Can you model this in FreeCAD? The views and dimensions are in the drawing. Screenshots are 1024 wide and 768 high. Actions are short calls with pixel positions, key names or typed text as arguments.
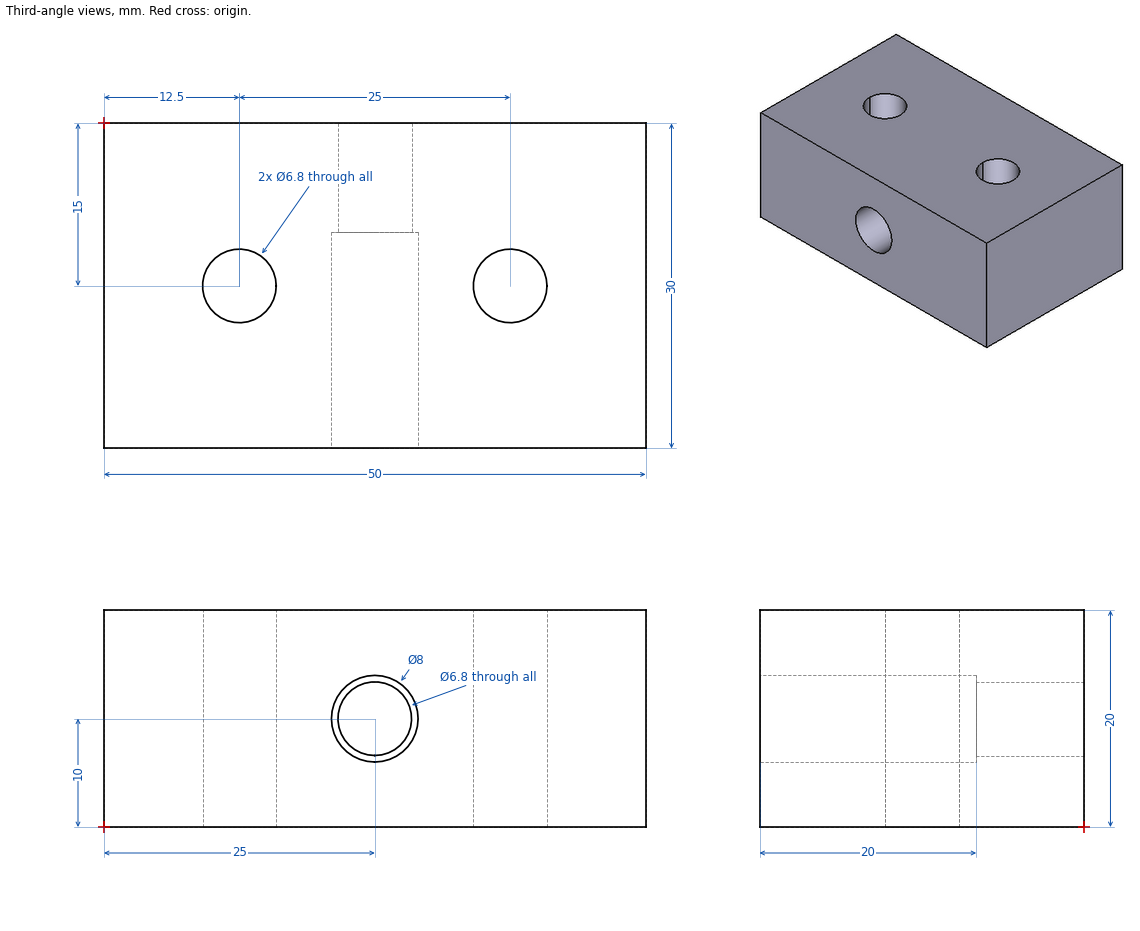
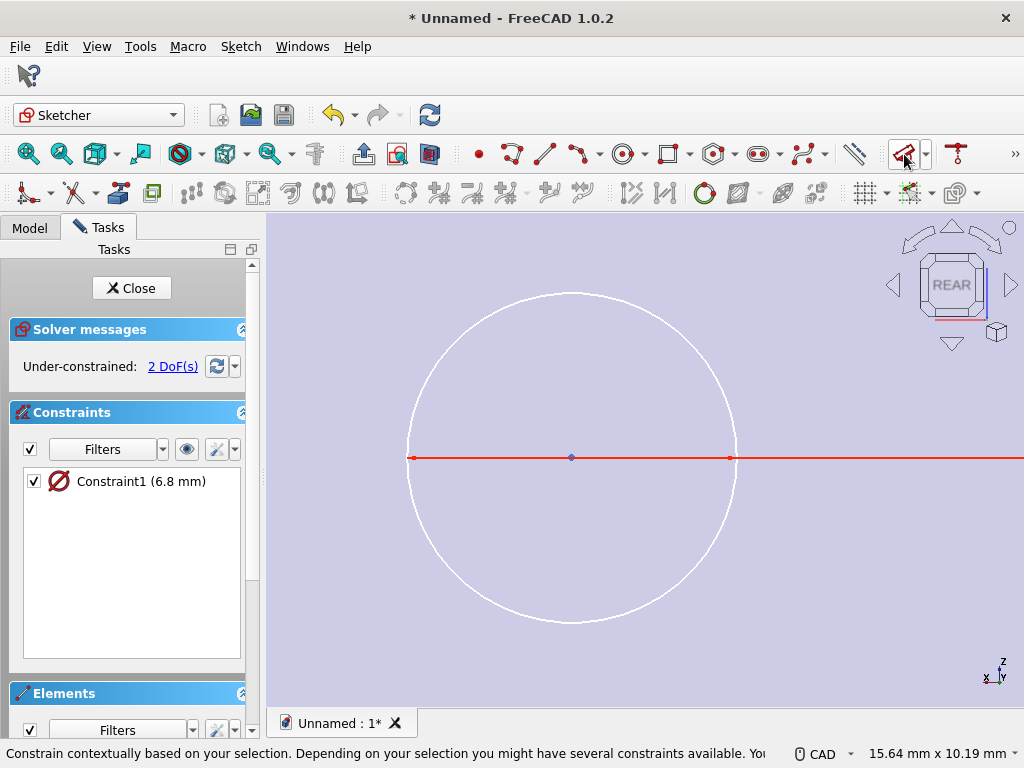
click(572, 458)
click(716, 424)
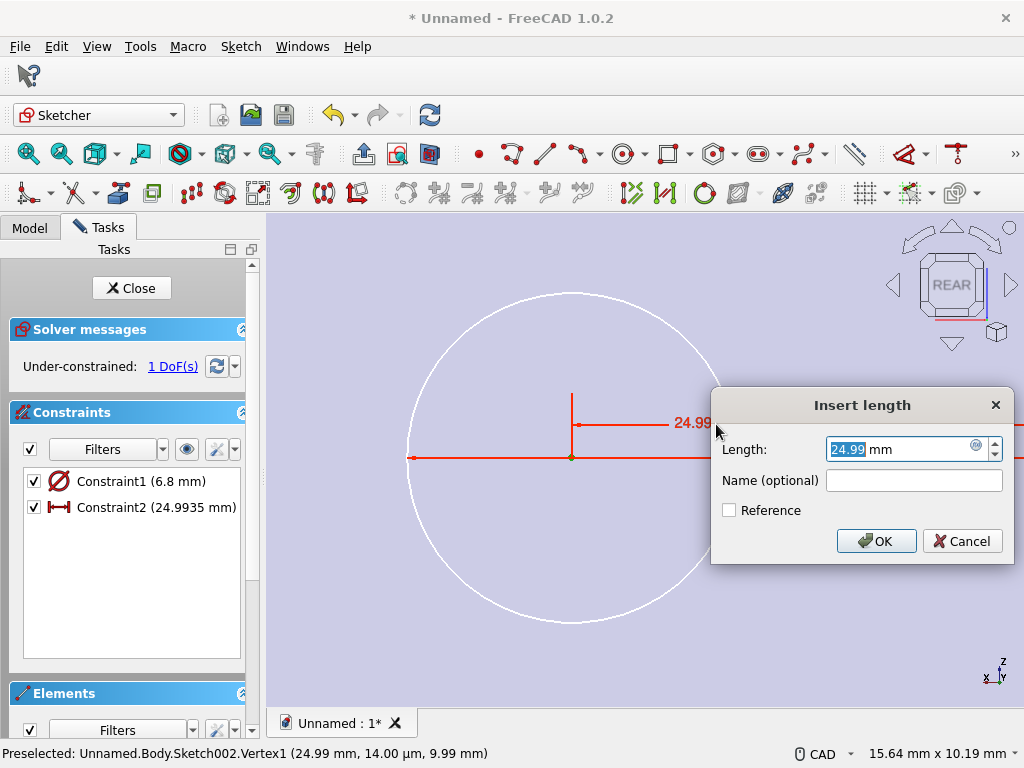
text(25)
key(Return)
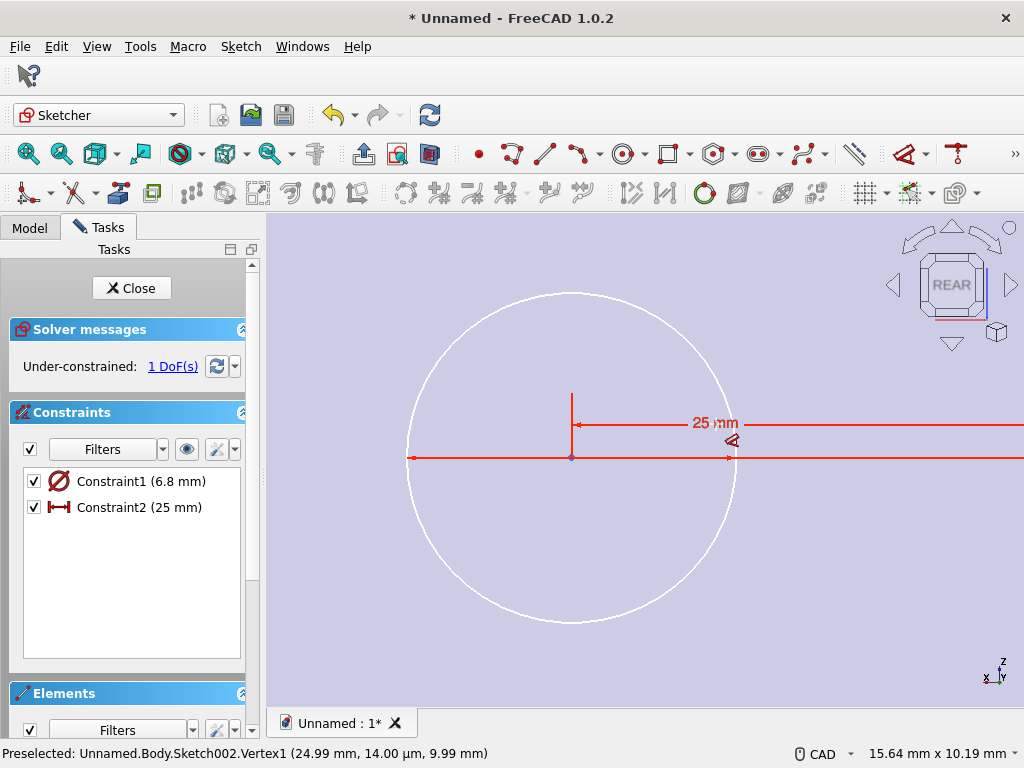
click(572, 458)
click(538, 568)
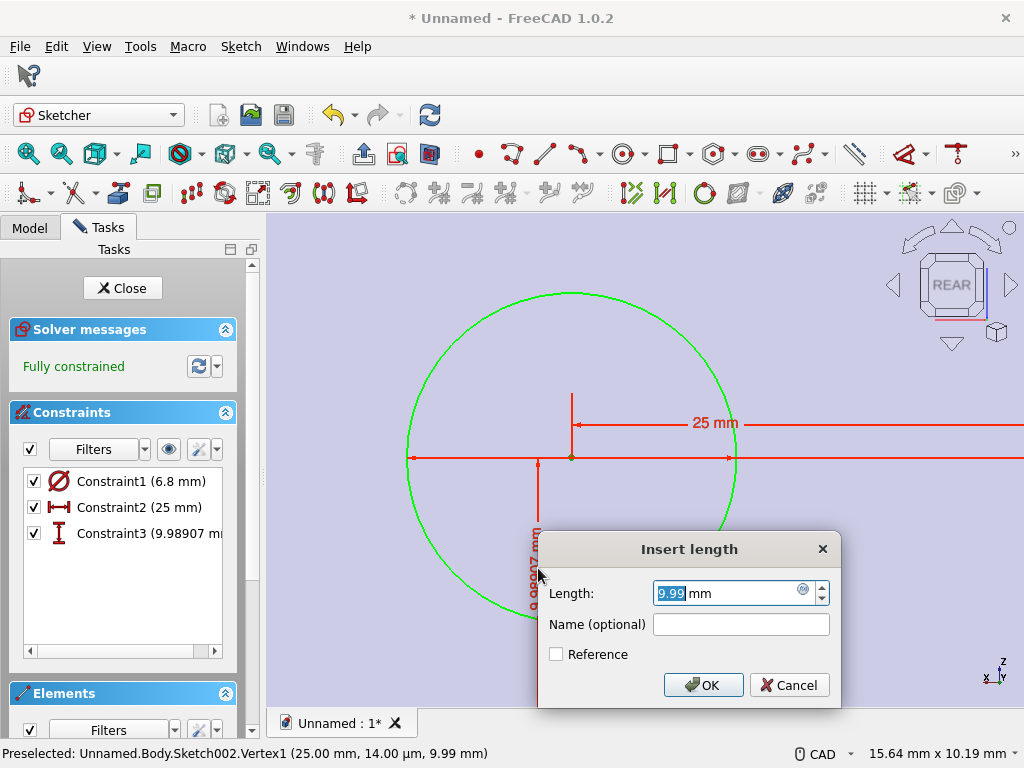
text(10)
key(Return)
key(Escape)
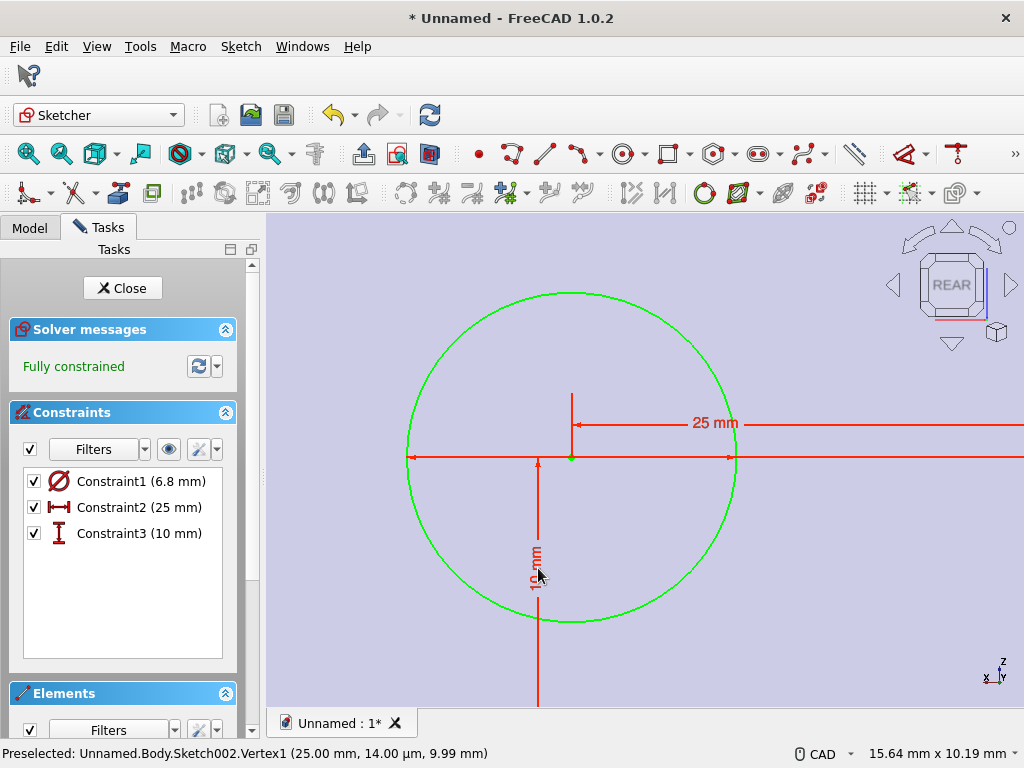
click(123, 288)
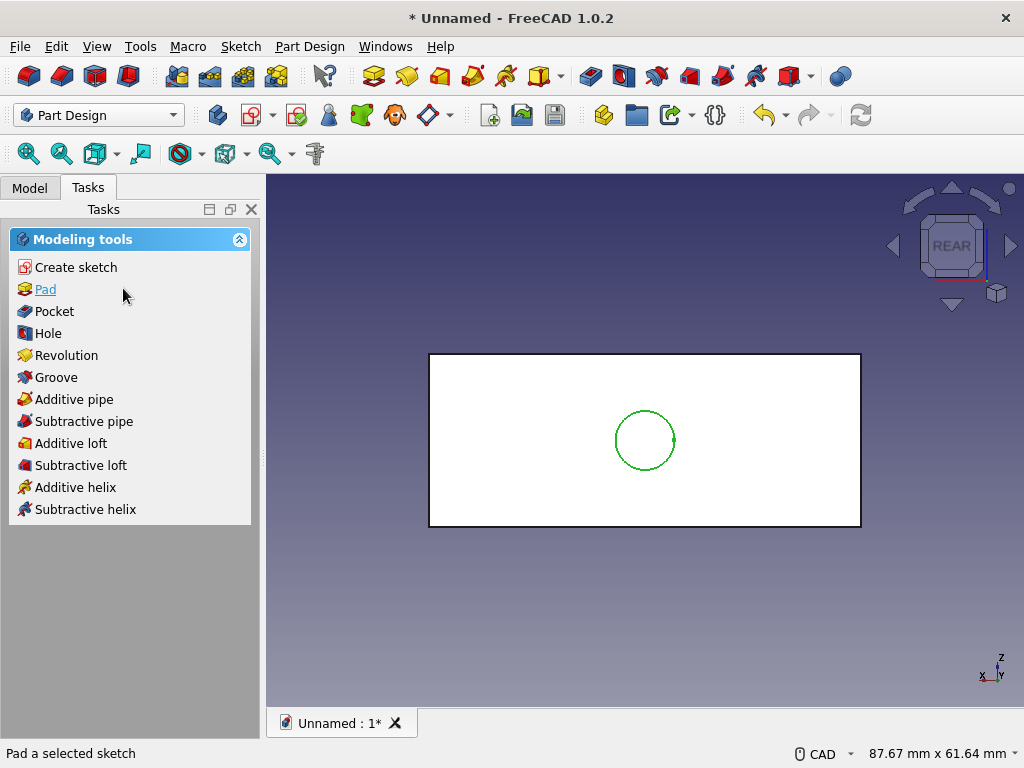
click(624, 76)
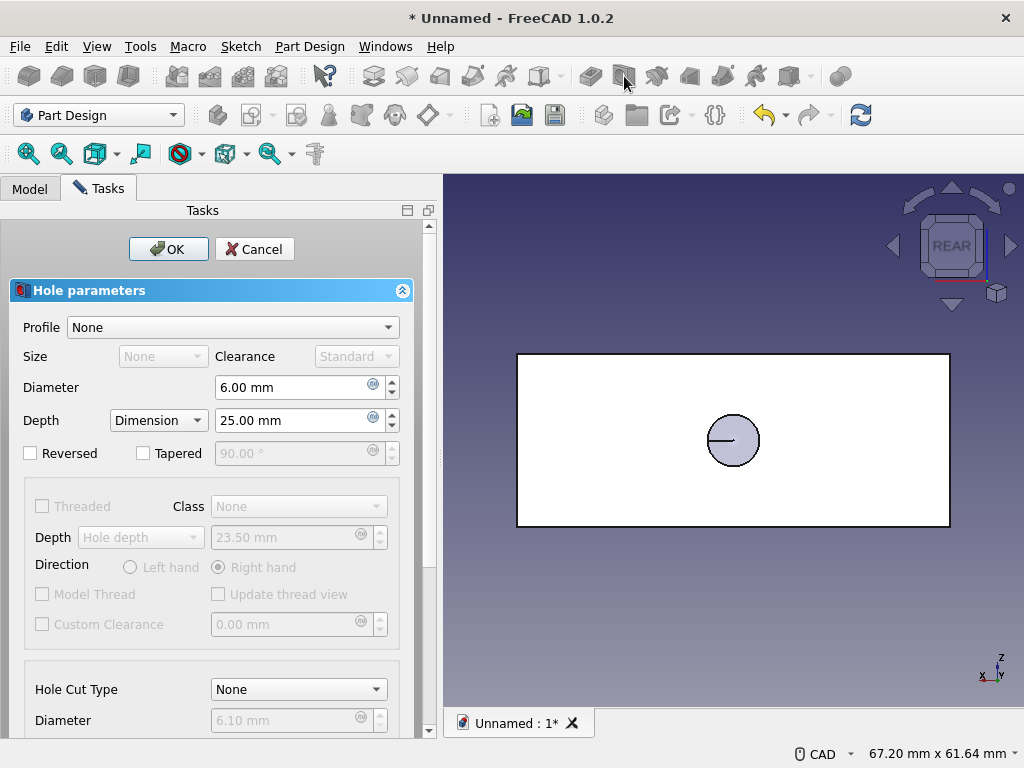
triple_click(300, 388)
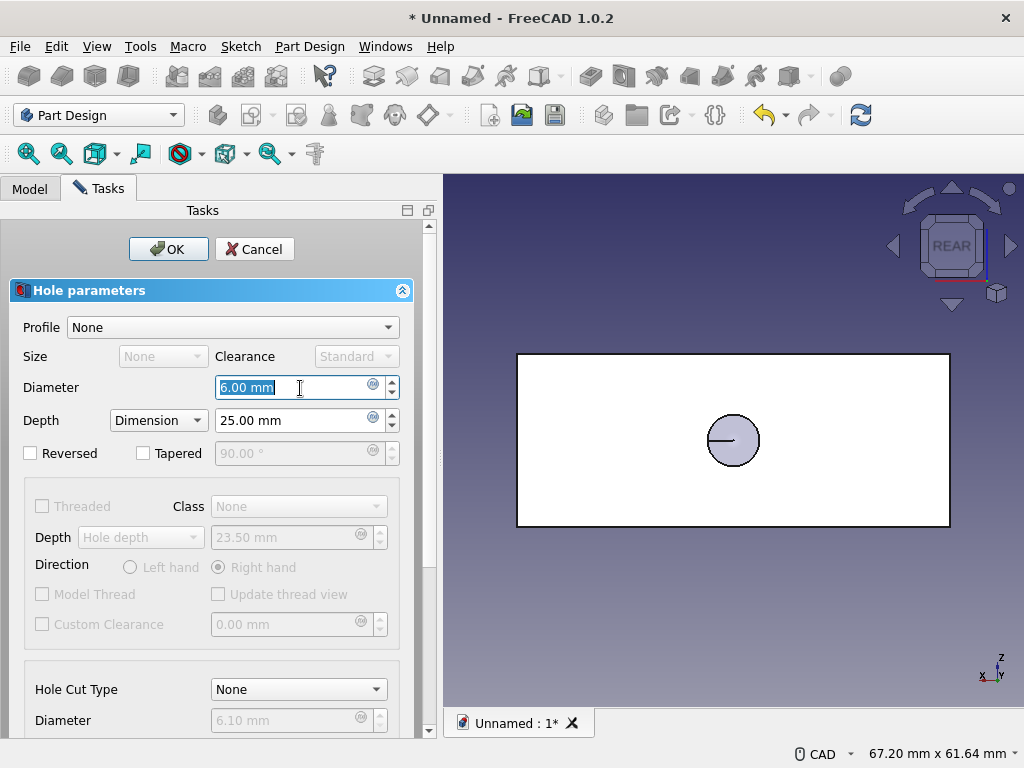
text(6.8)
key(Tab)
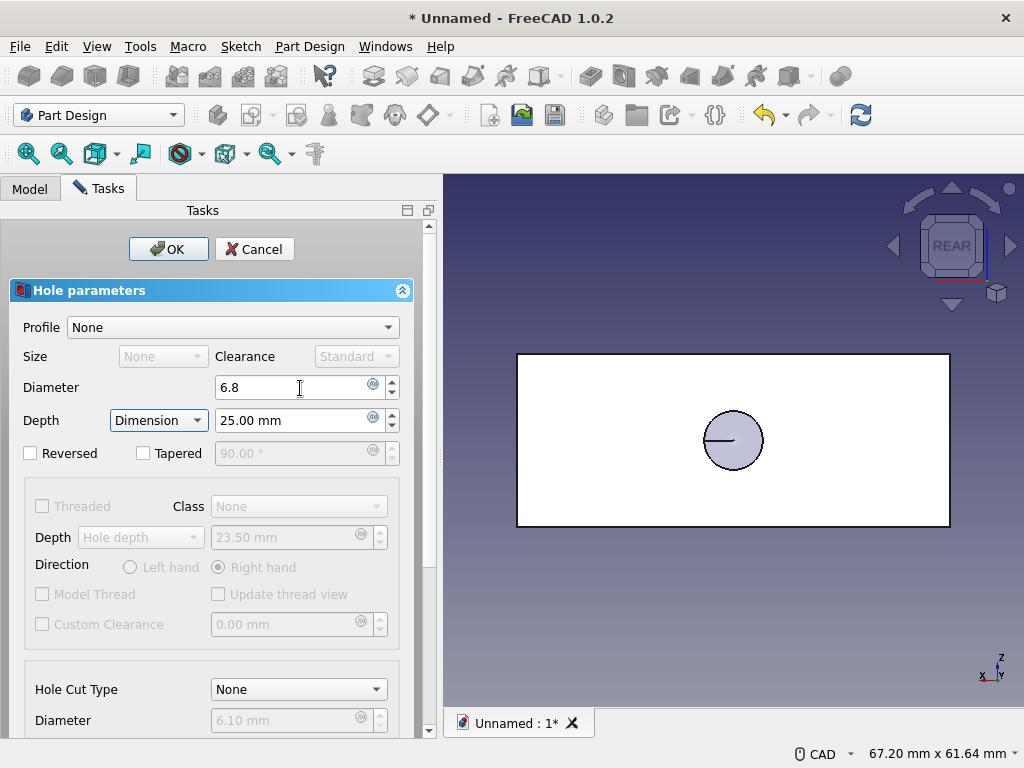
click(160, 420)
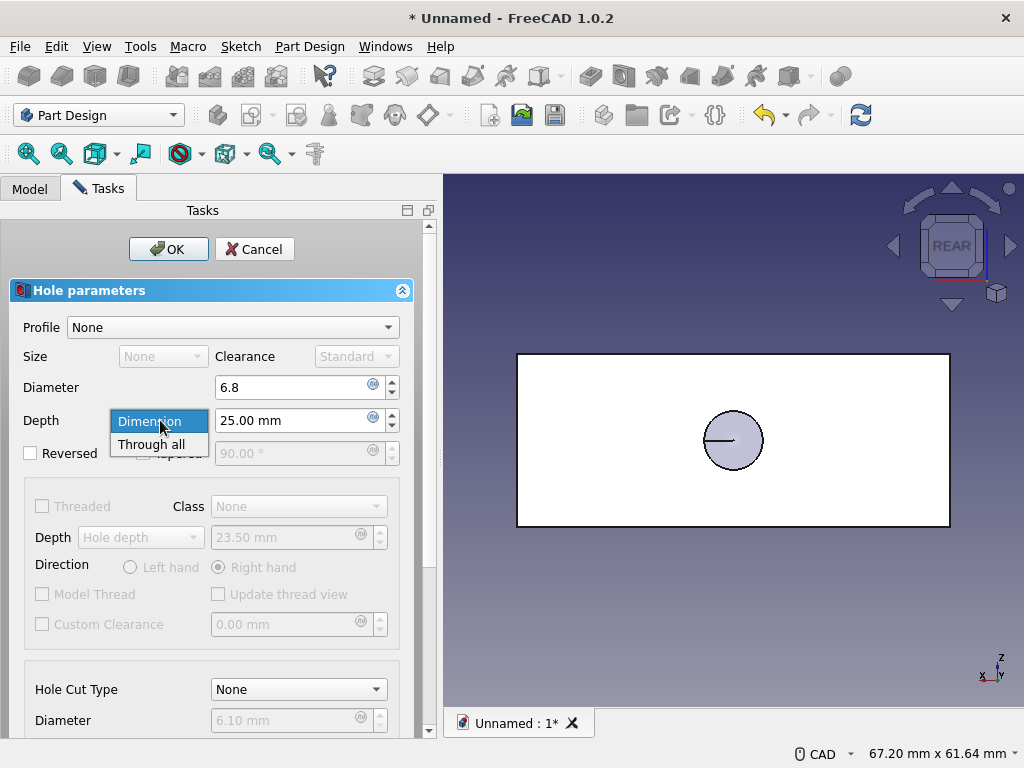
click(158, 444)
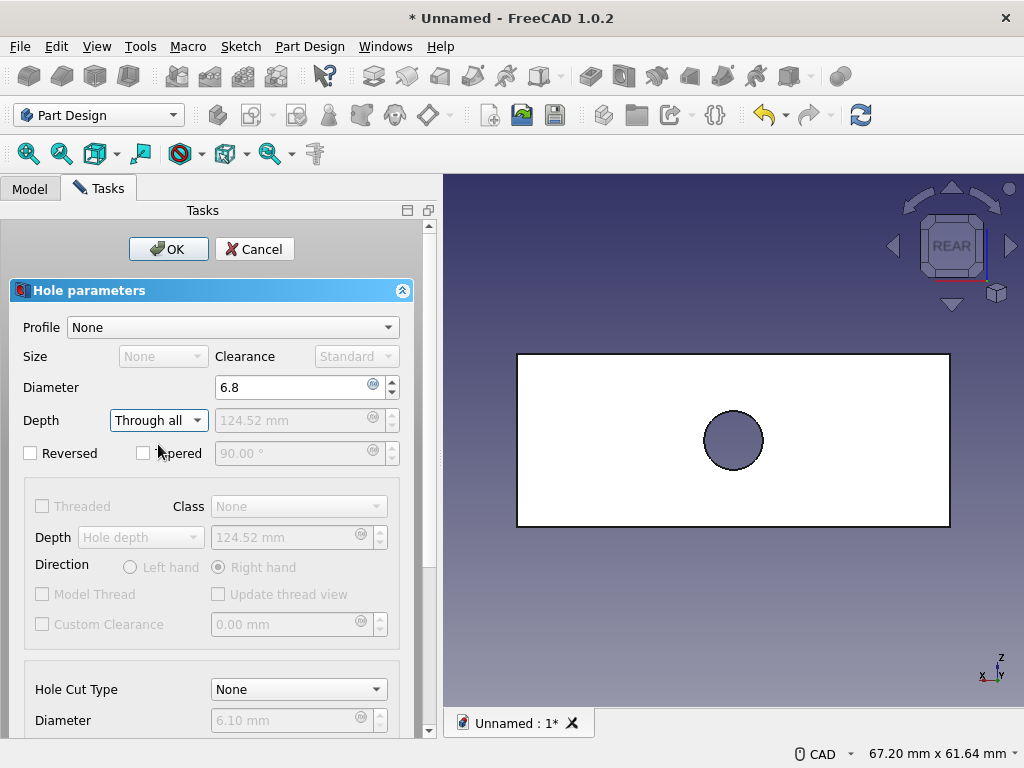
click(169, 249)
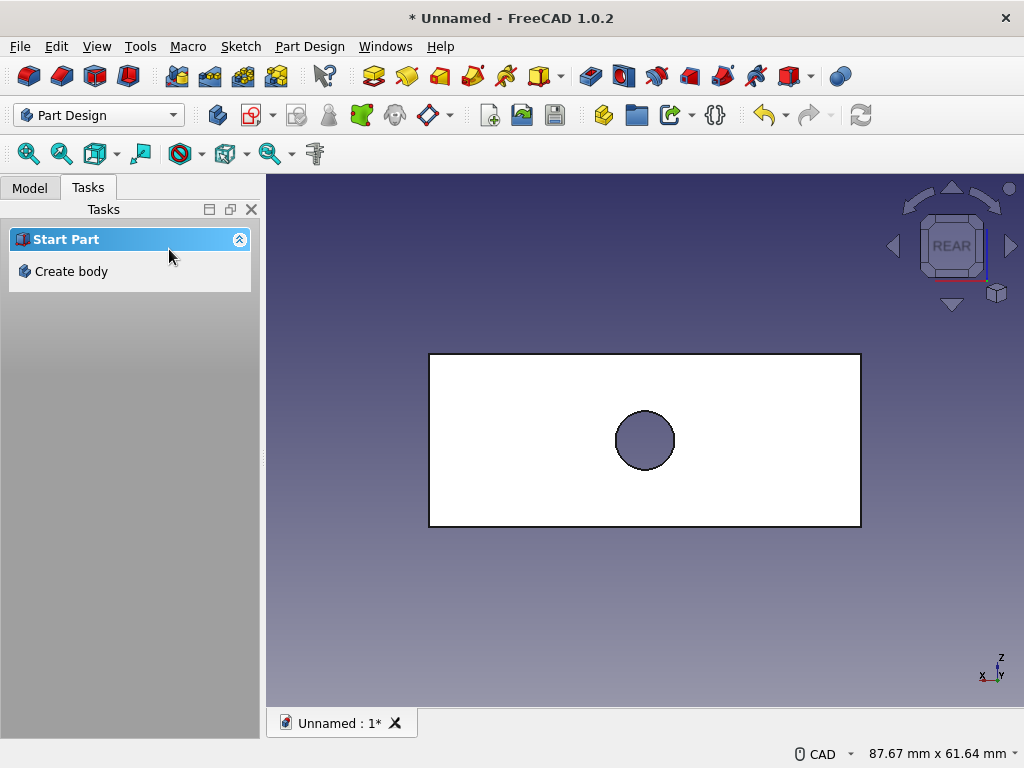
key(0)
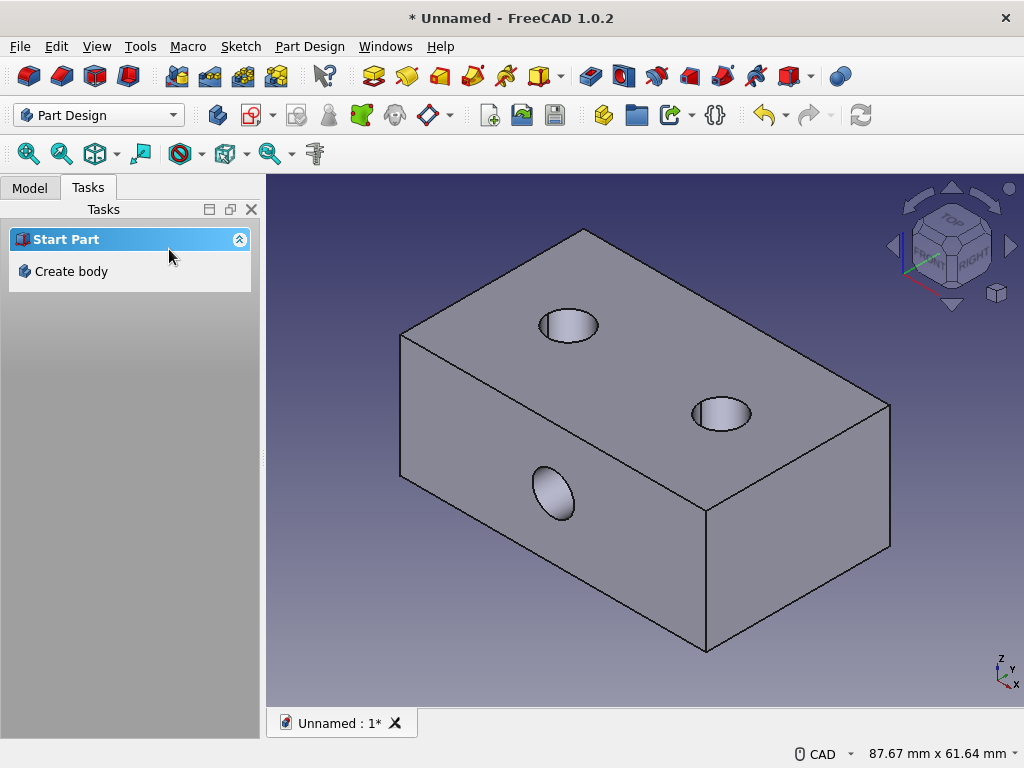
click(641, 543)